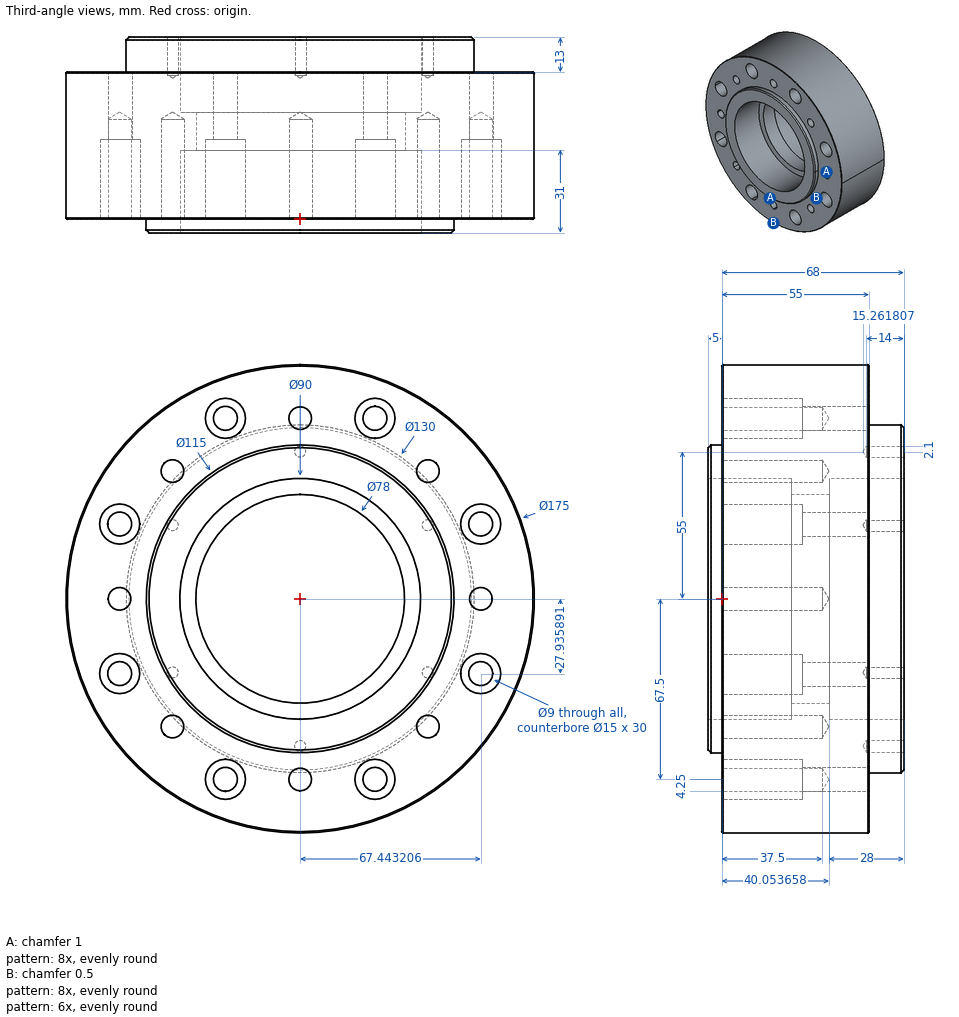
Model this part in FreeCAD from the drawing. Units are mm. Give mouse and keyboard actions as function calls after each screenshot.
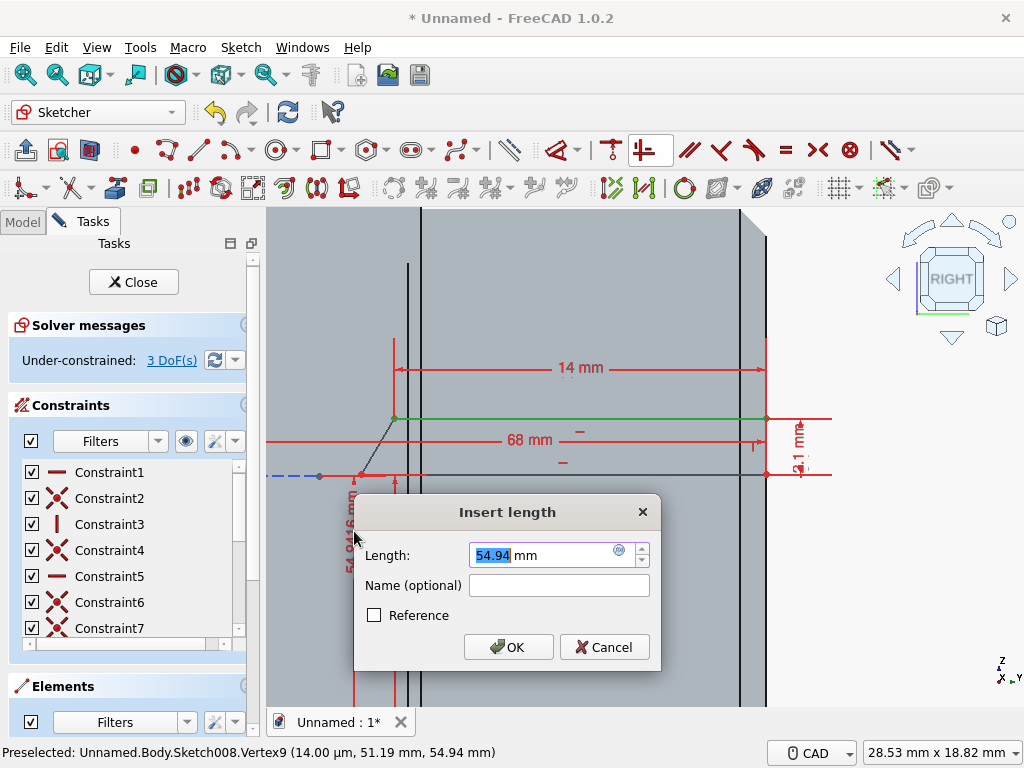
text(55)
key(Return)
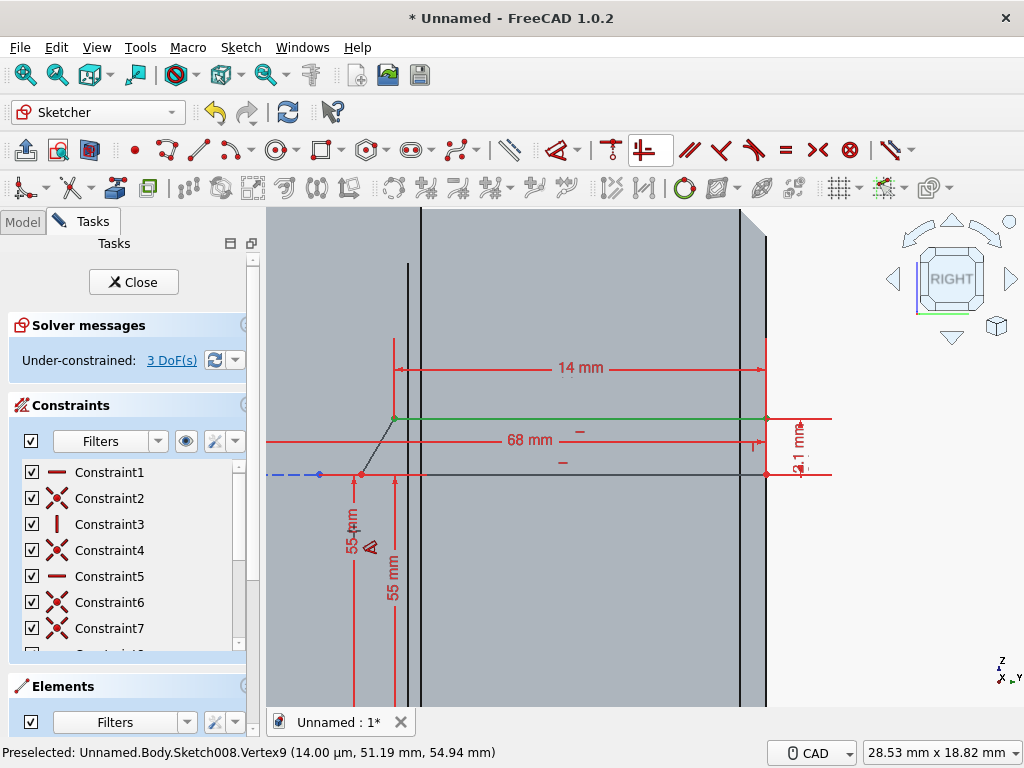
click(483, 475)
click(564, 509)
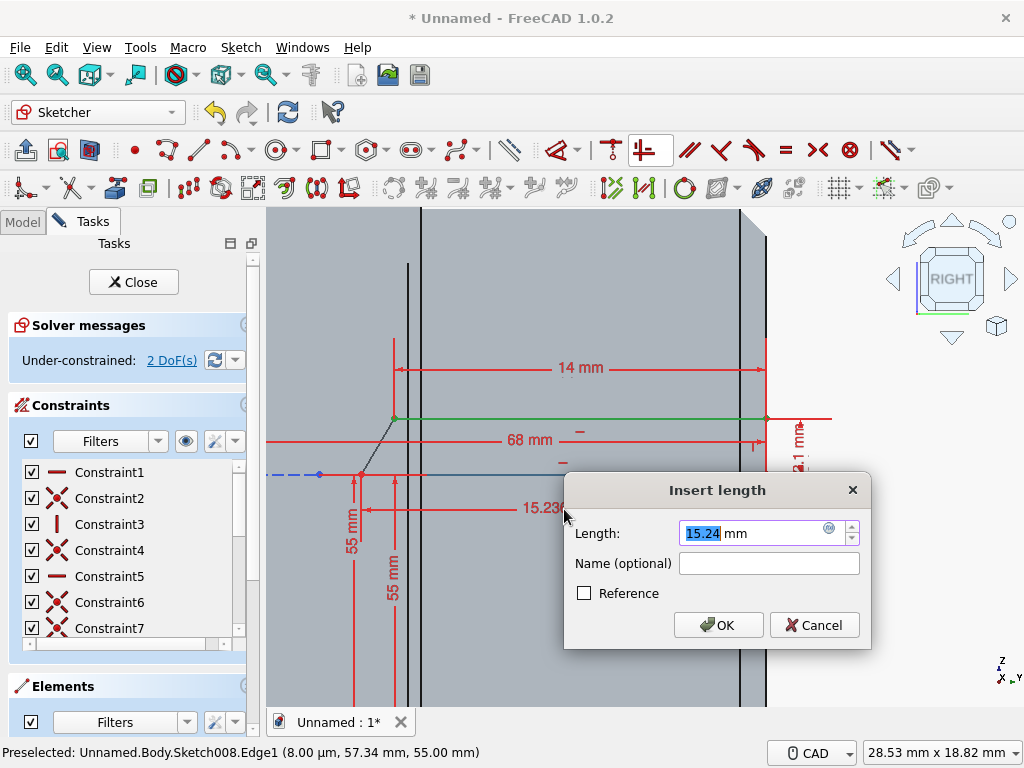
text(15.261807)
key(Return)
key(Escape)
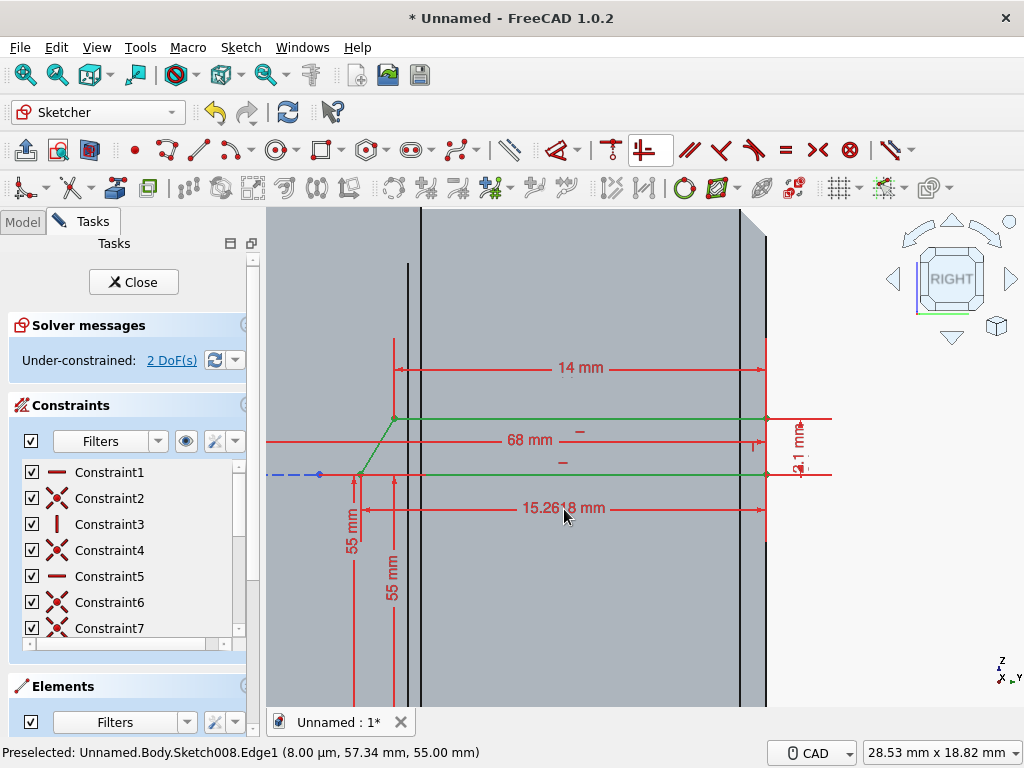
click(134, 282)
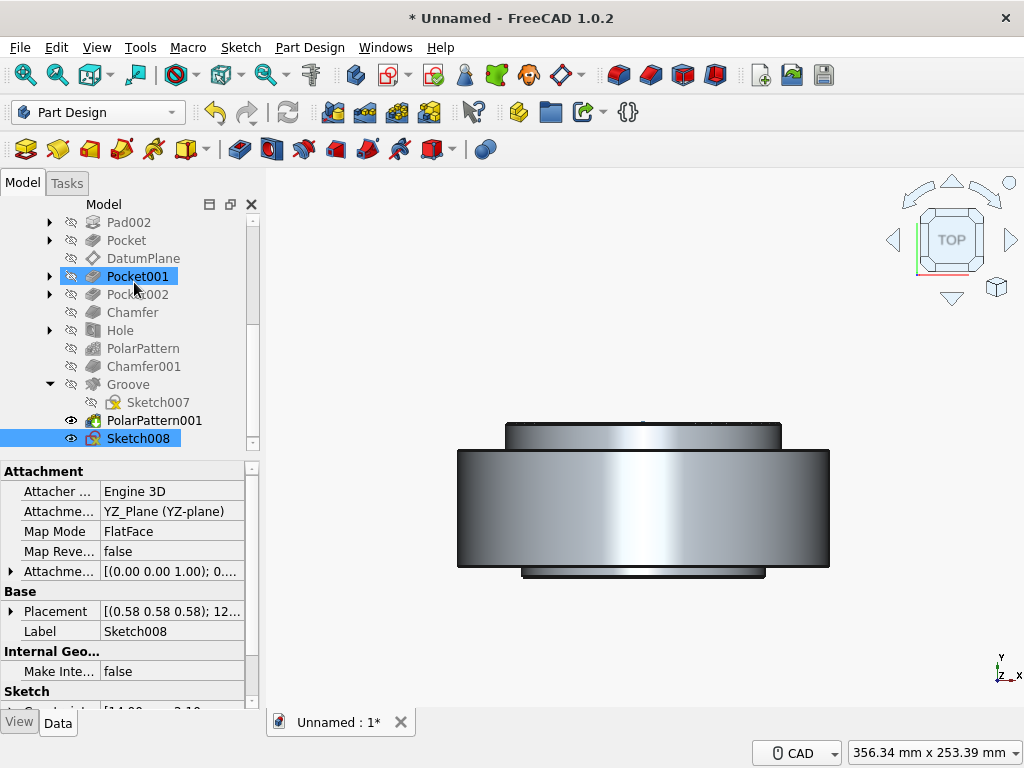
click(304, 150)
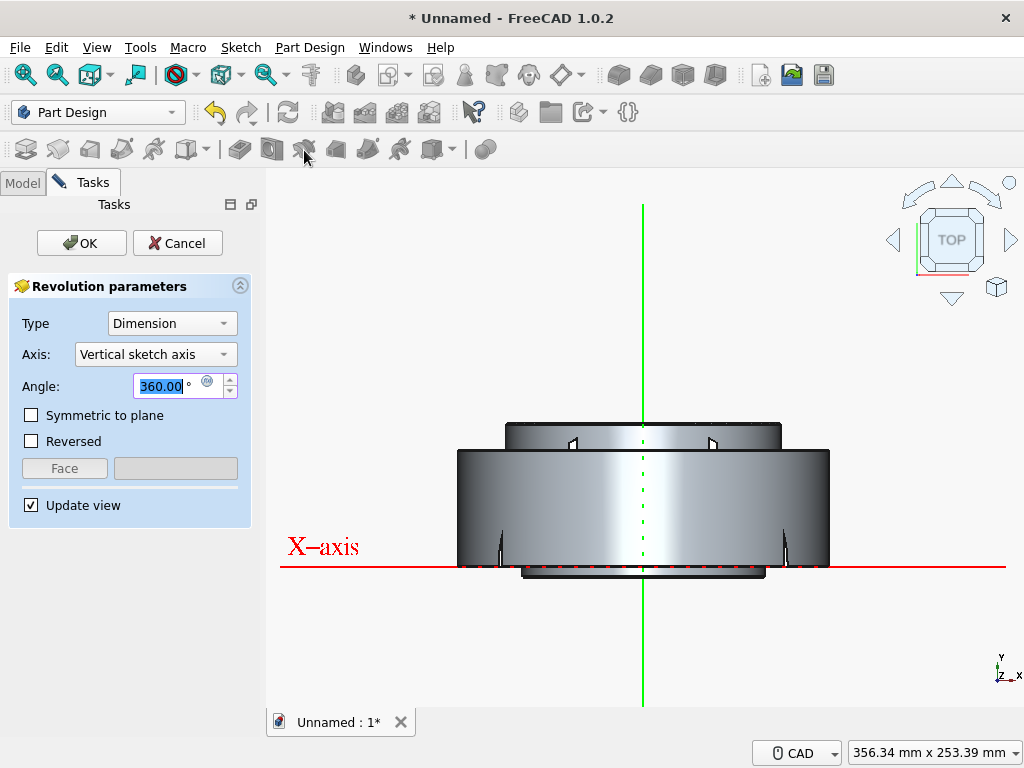
click(156, 354)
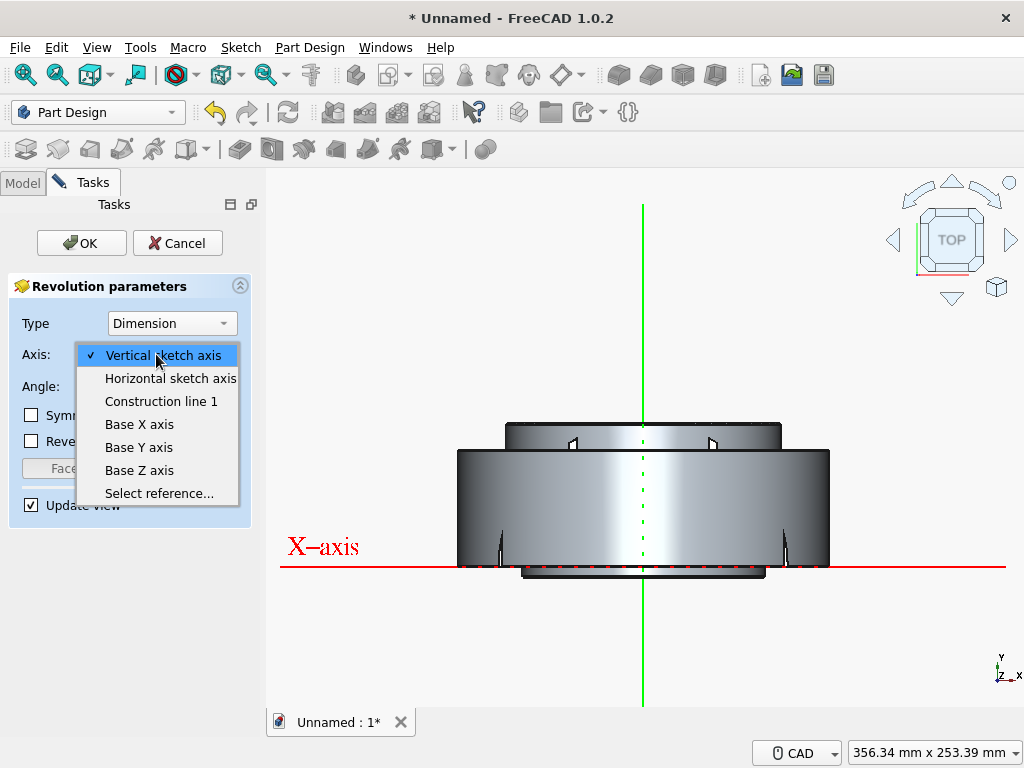
click(156, 402)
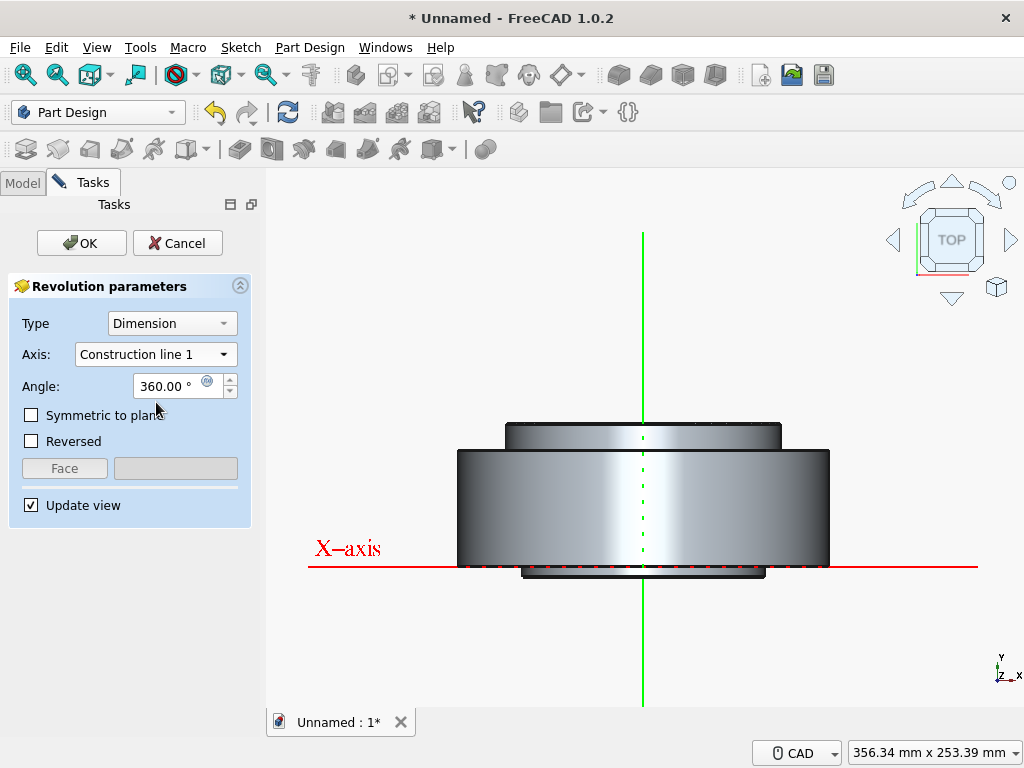
click(82, 243)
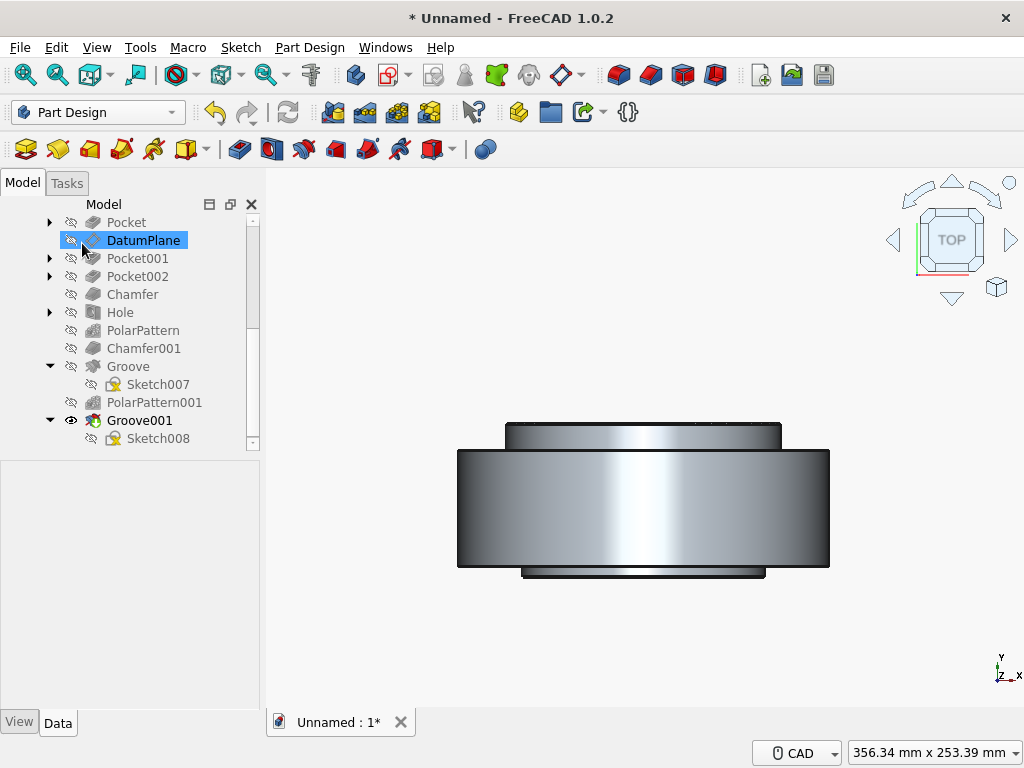
click(116, 420)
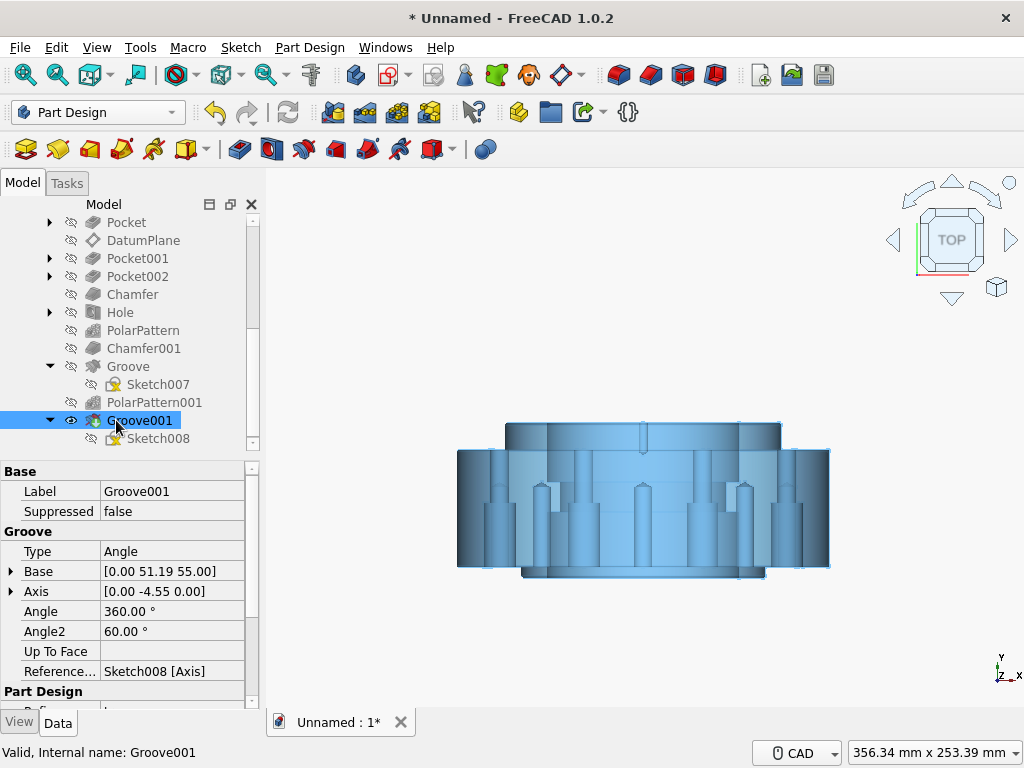
click(398, 112)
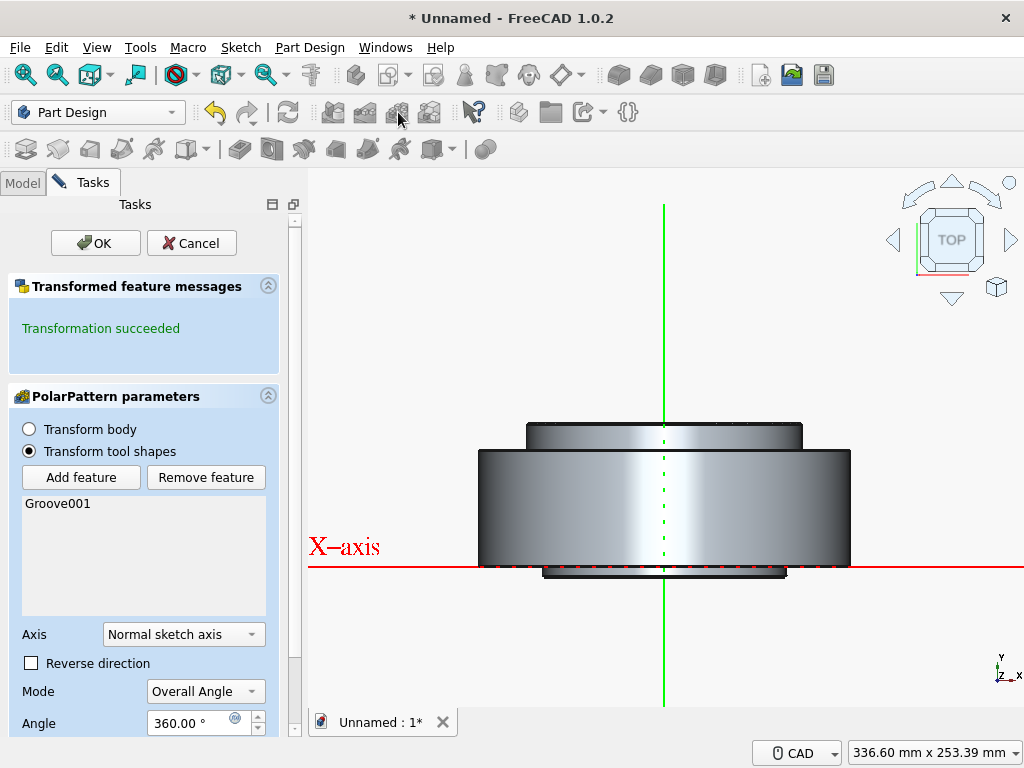
click(184, 634)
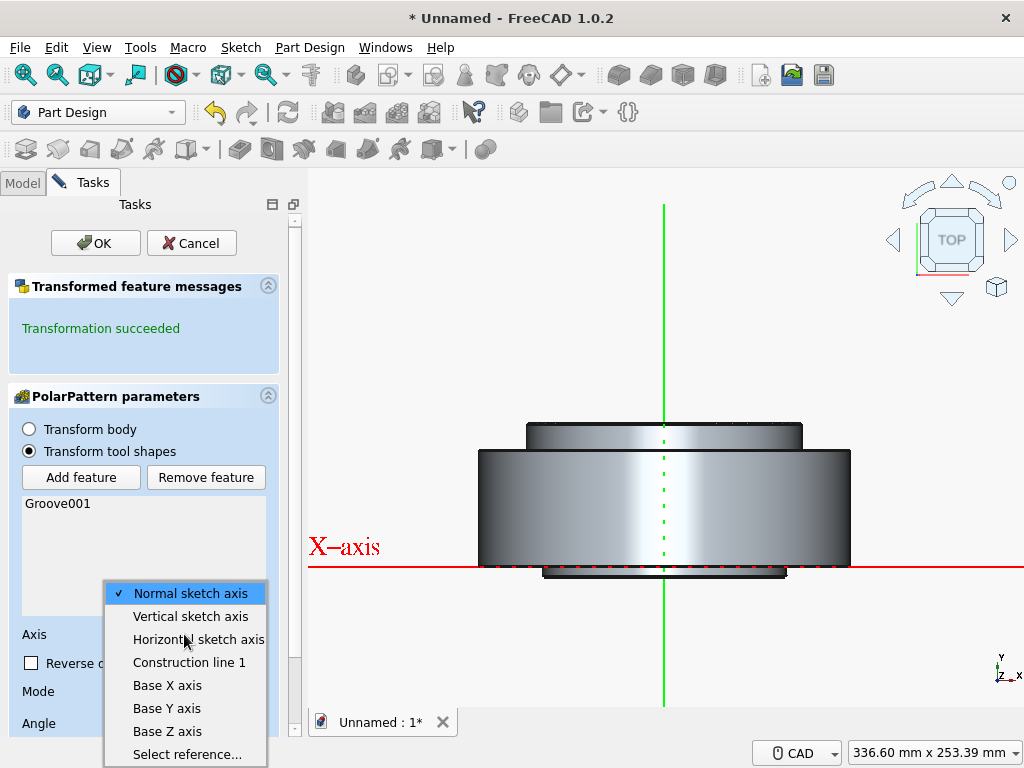
click(184, 708)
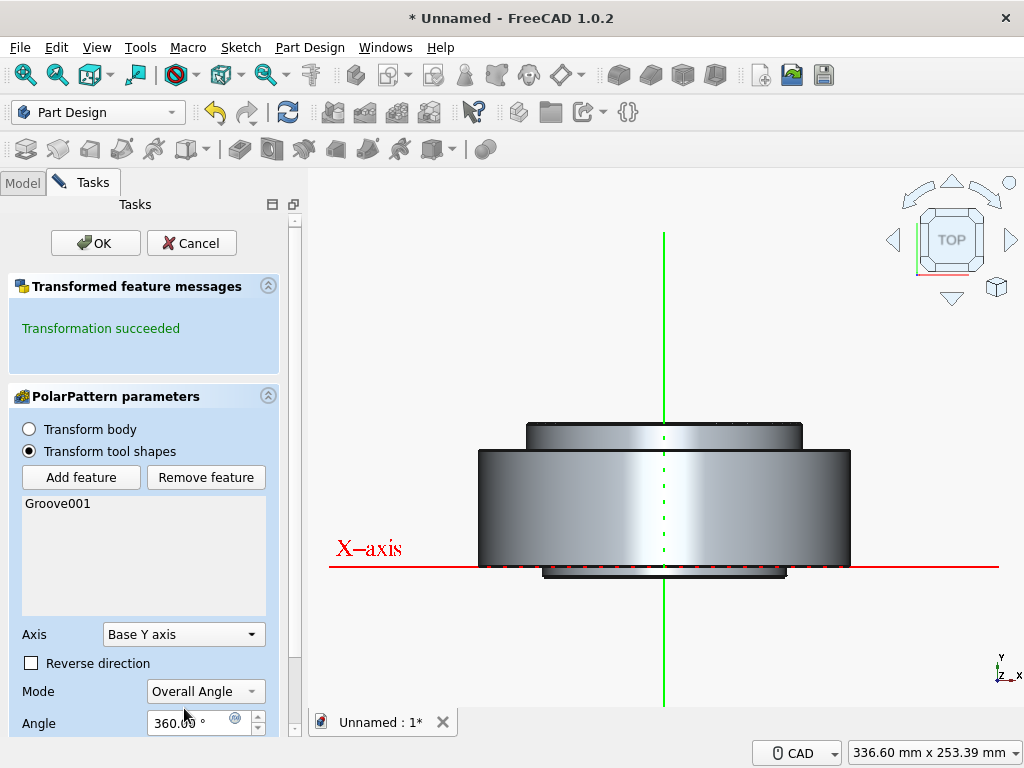
scroll(295, 475, down, 2)